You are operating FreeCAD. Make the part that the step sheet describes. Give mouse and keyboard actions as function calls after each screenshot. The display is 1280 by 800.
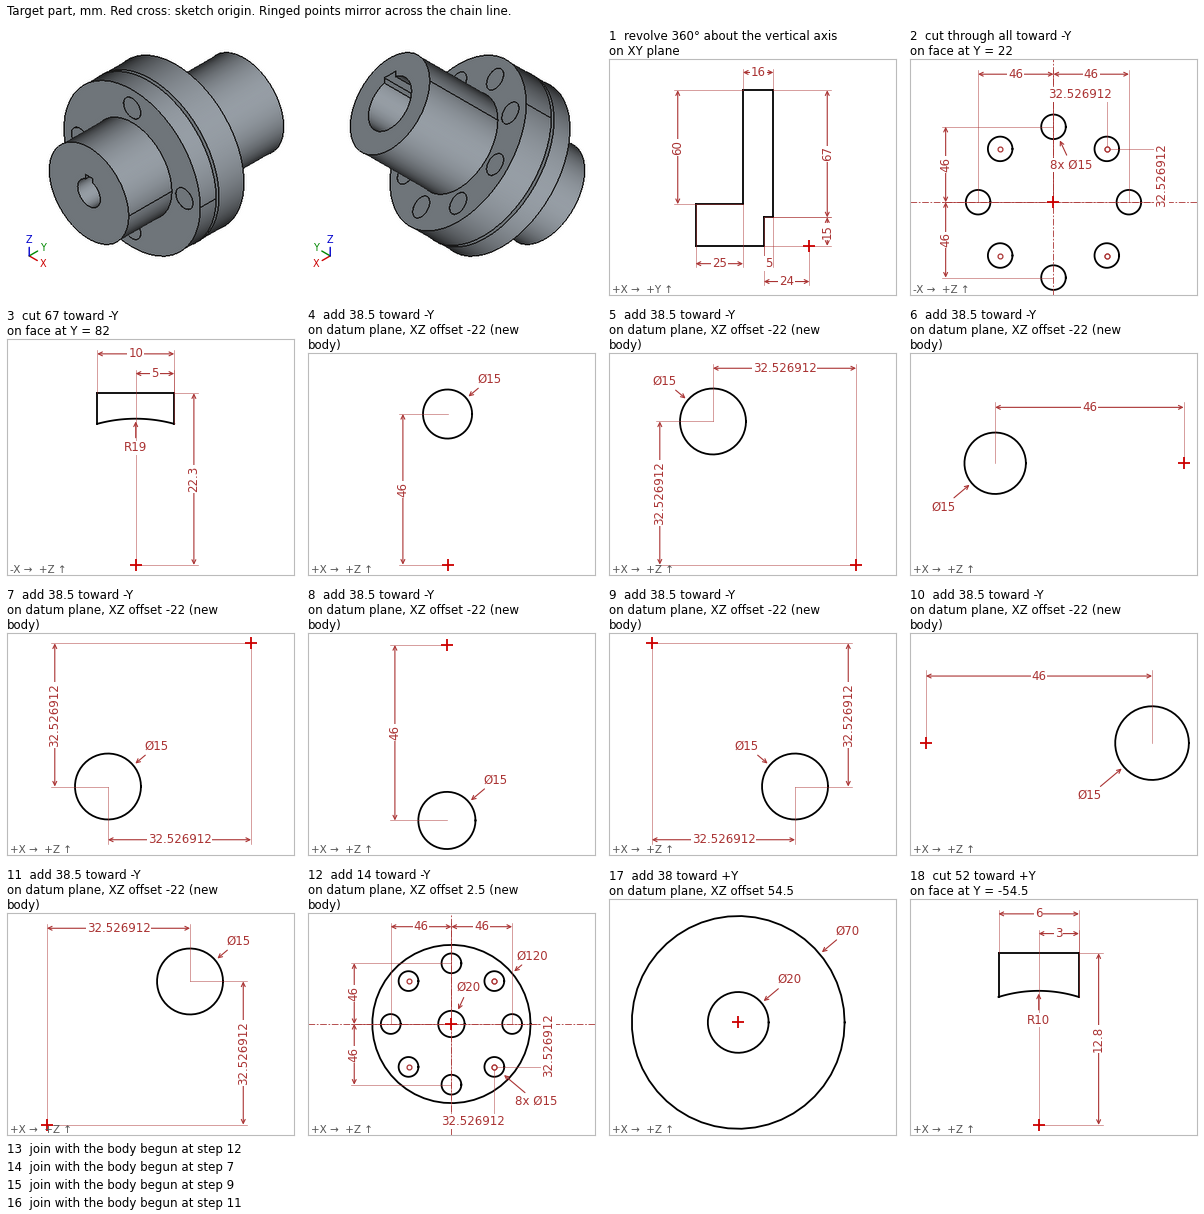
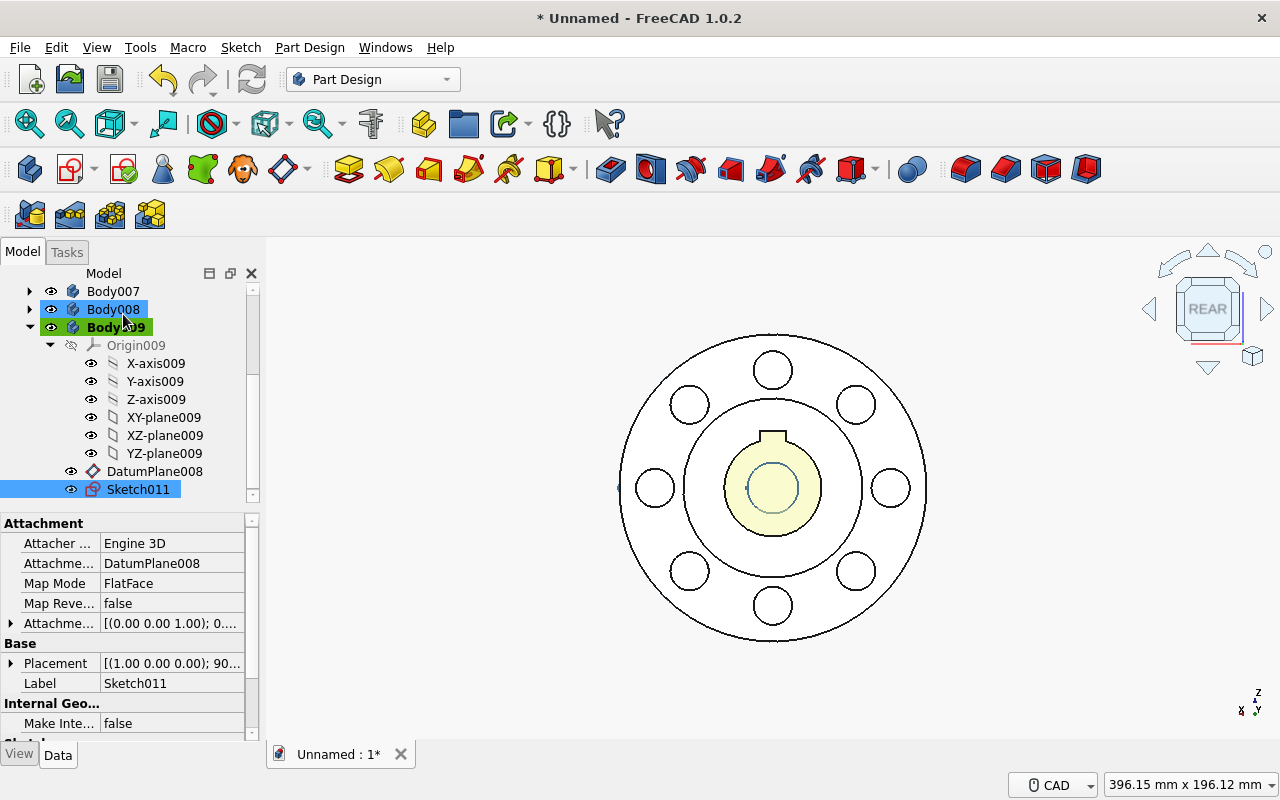
click(350, 170)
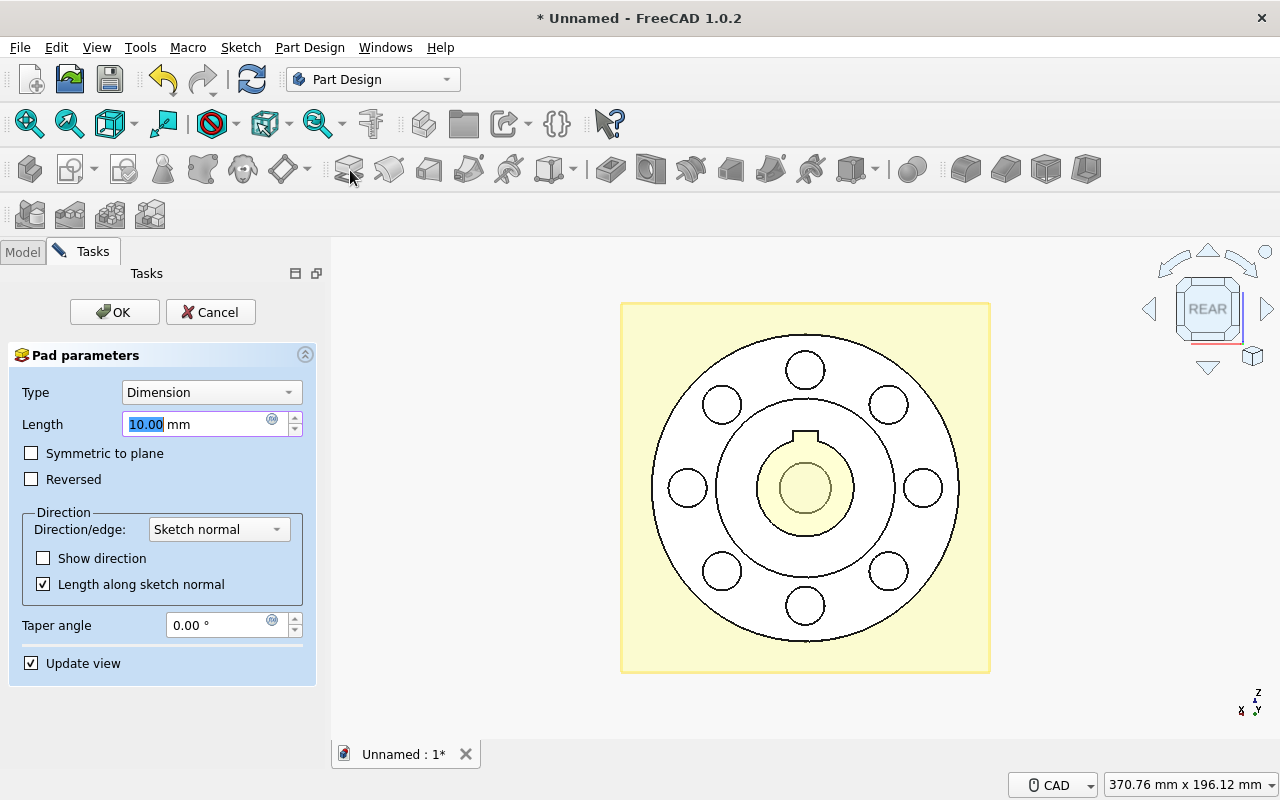
text(14)
key(Tab)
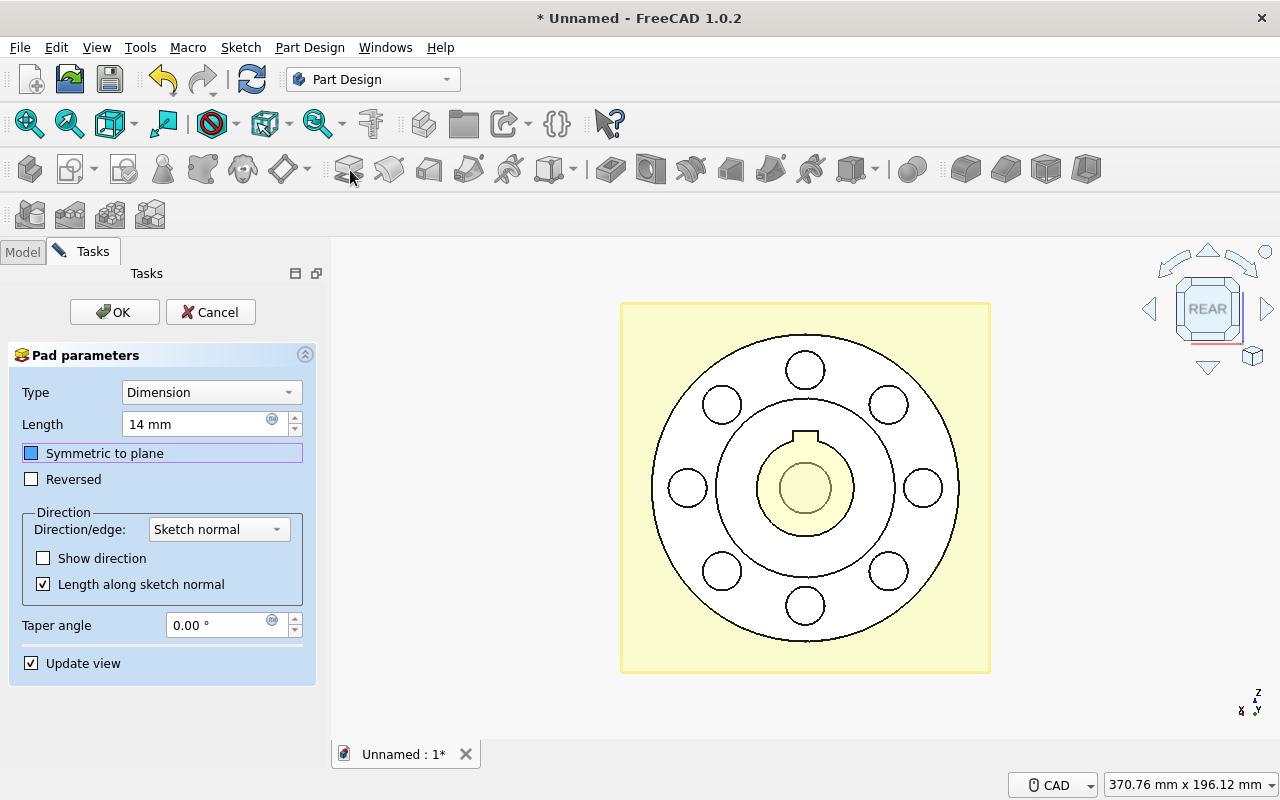
click(115, 312)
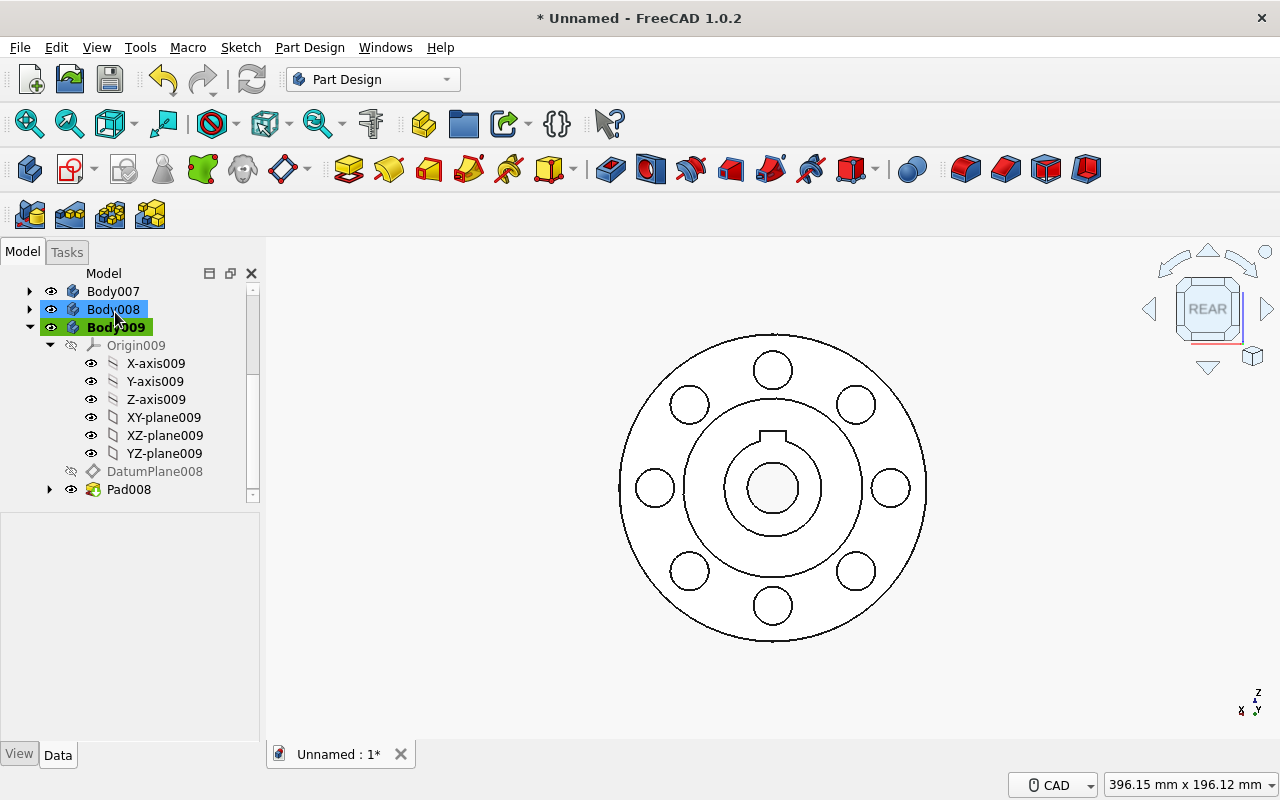
scroll(120, 395, down, 3)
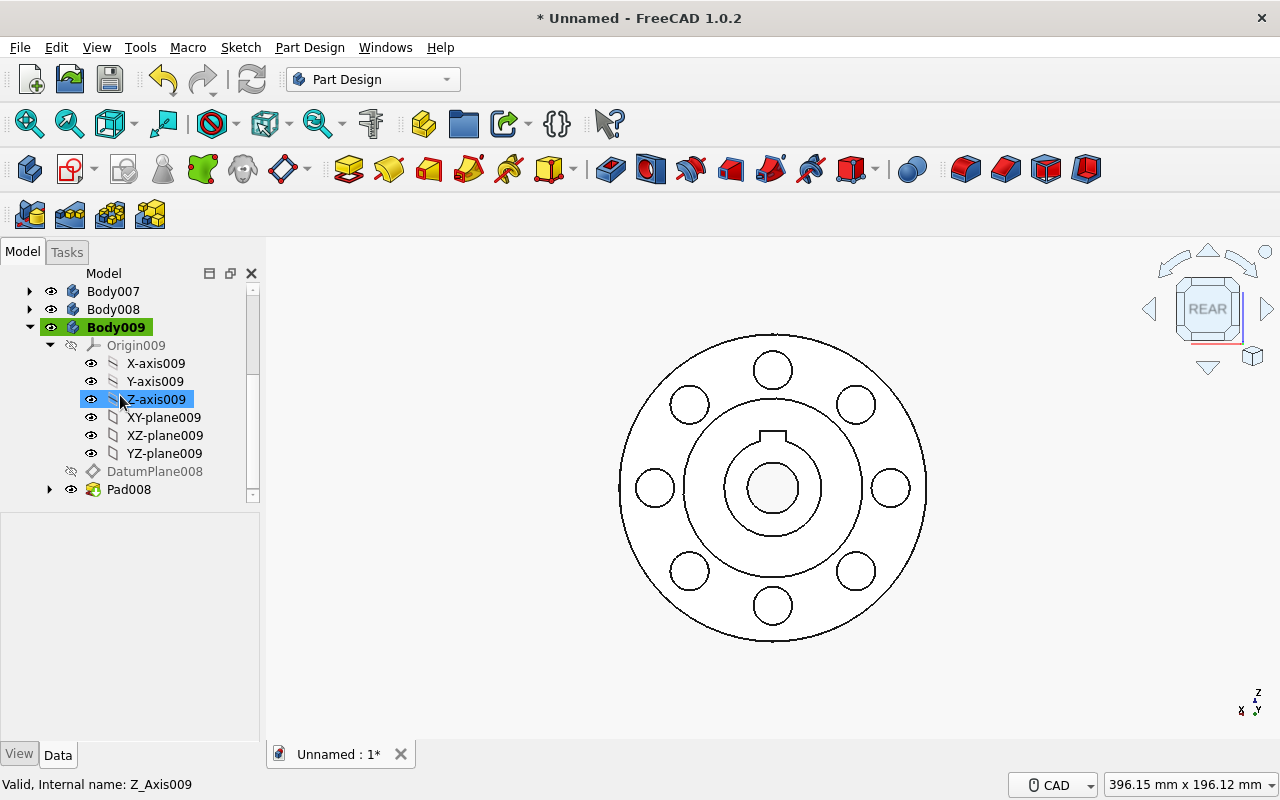
scroll(120, 395, up, 15)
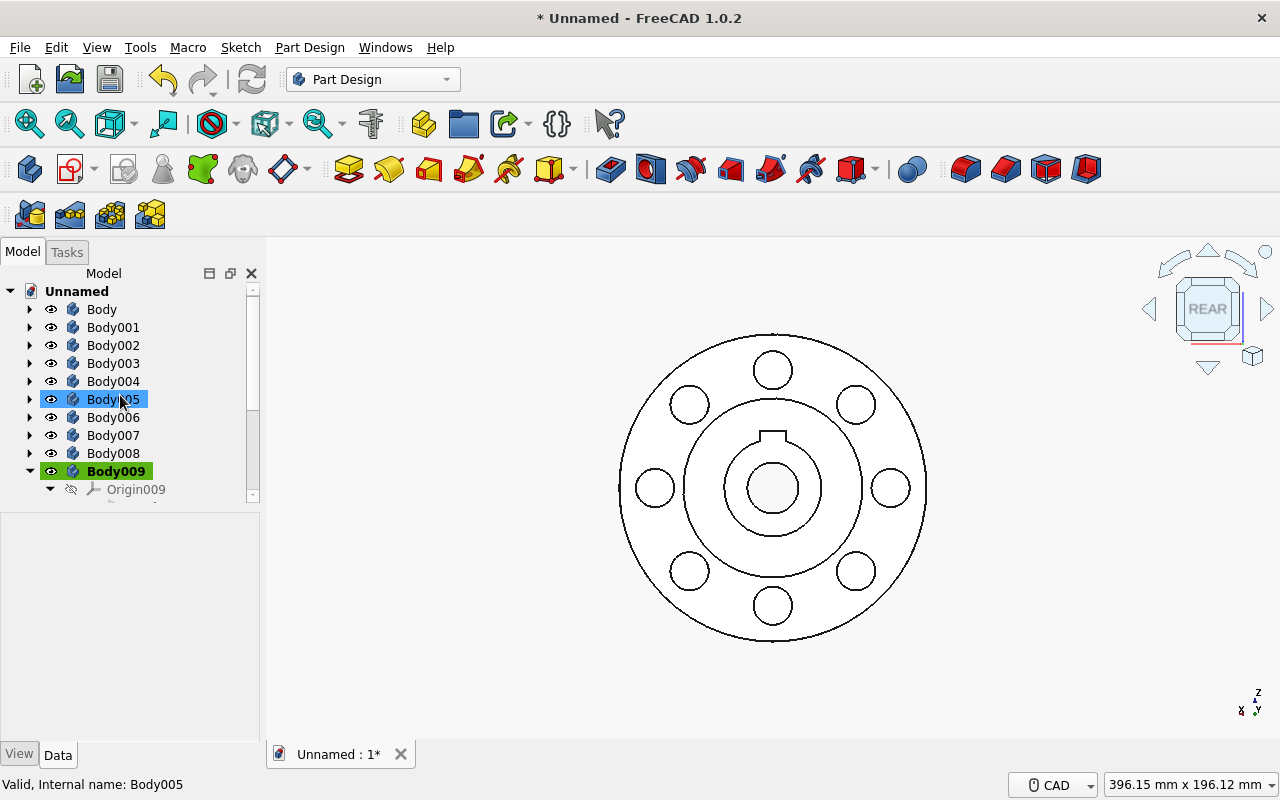
double_click(96, 345)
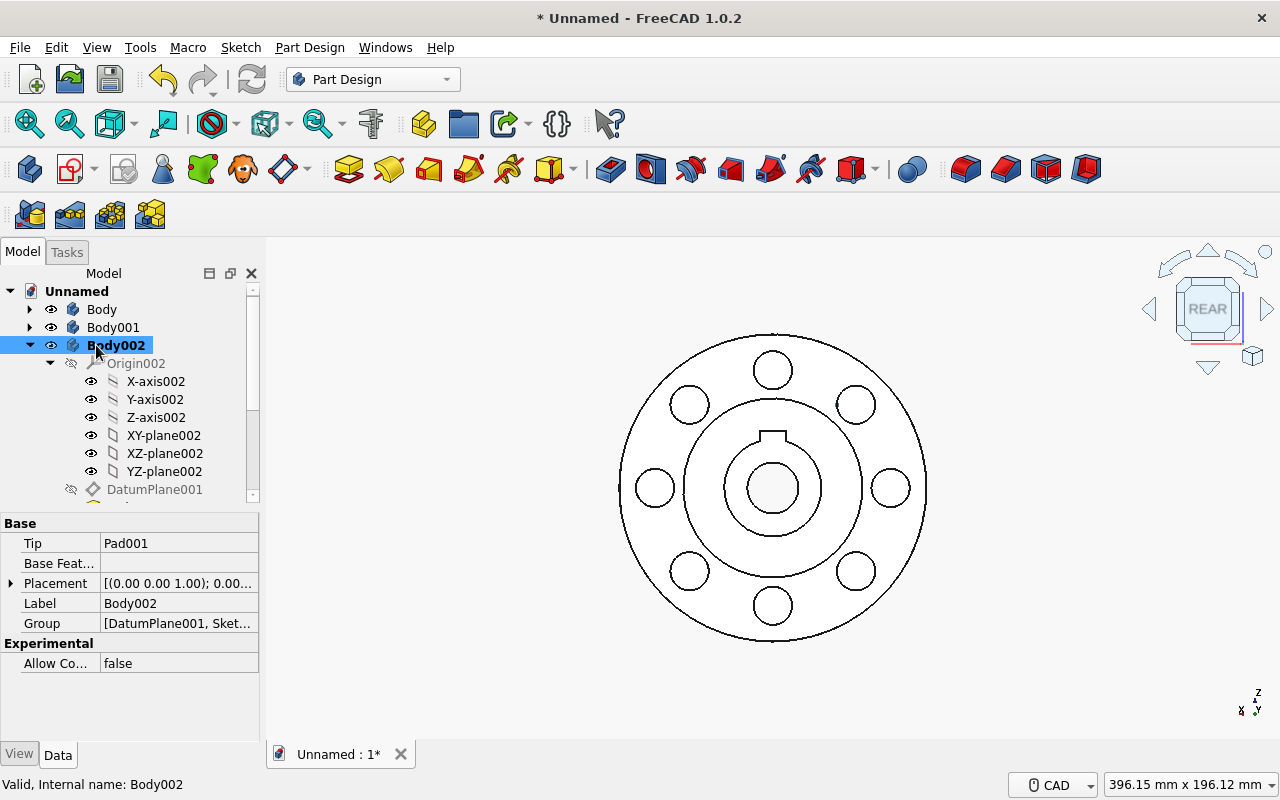
scroll(100, 395, down, 3)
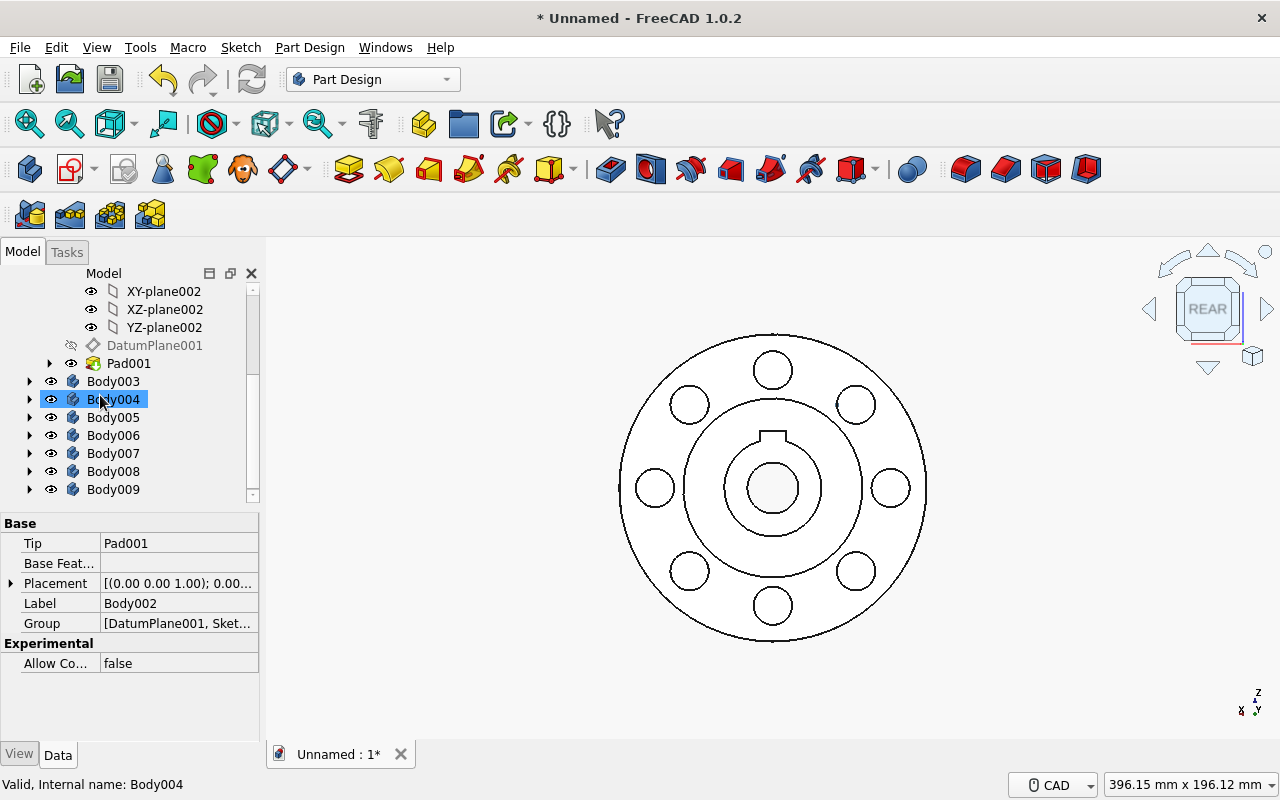
click(96, 489)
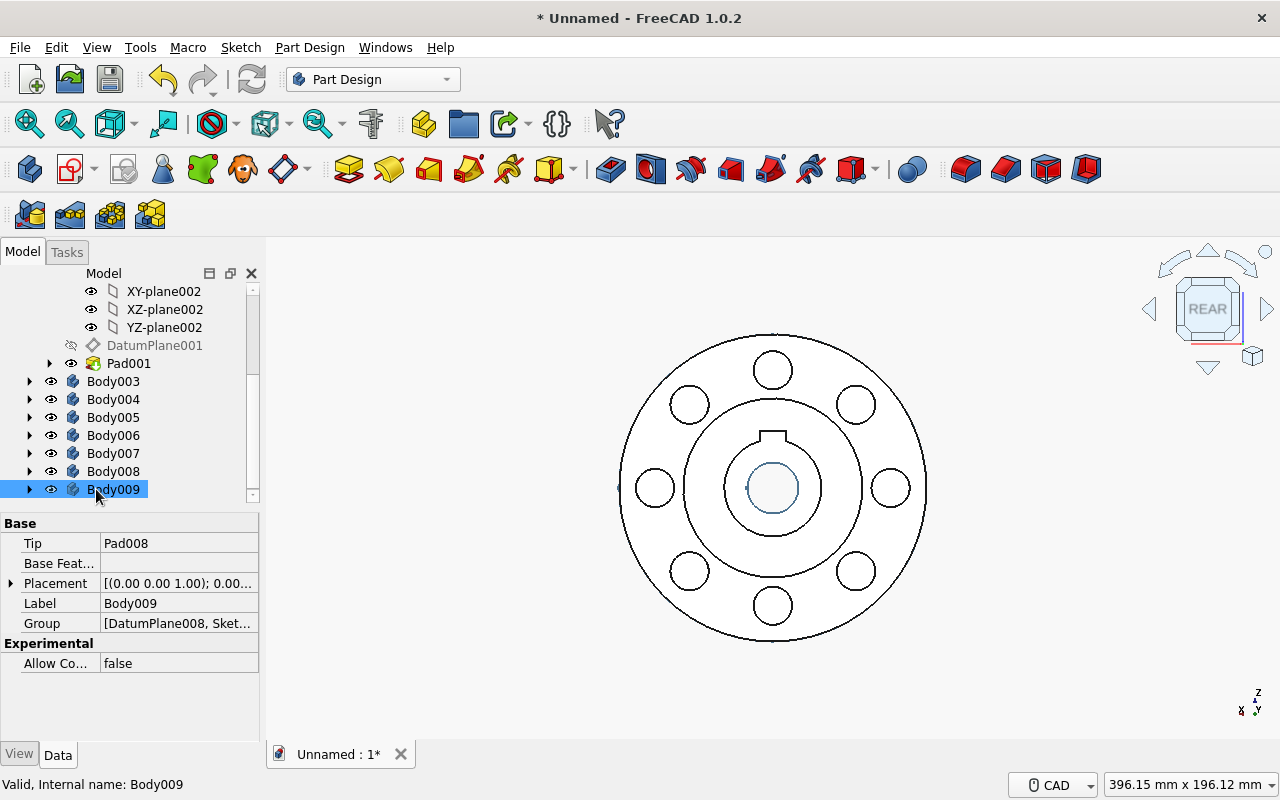
click(914, 170)